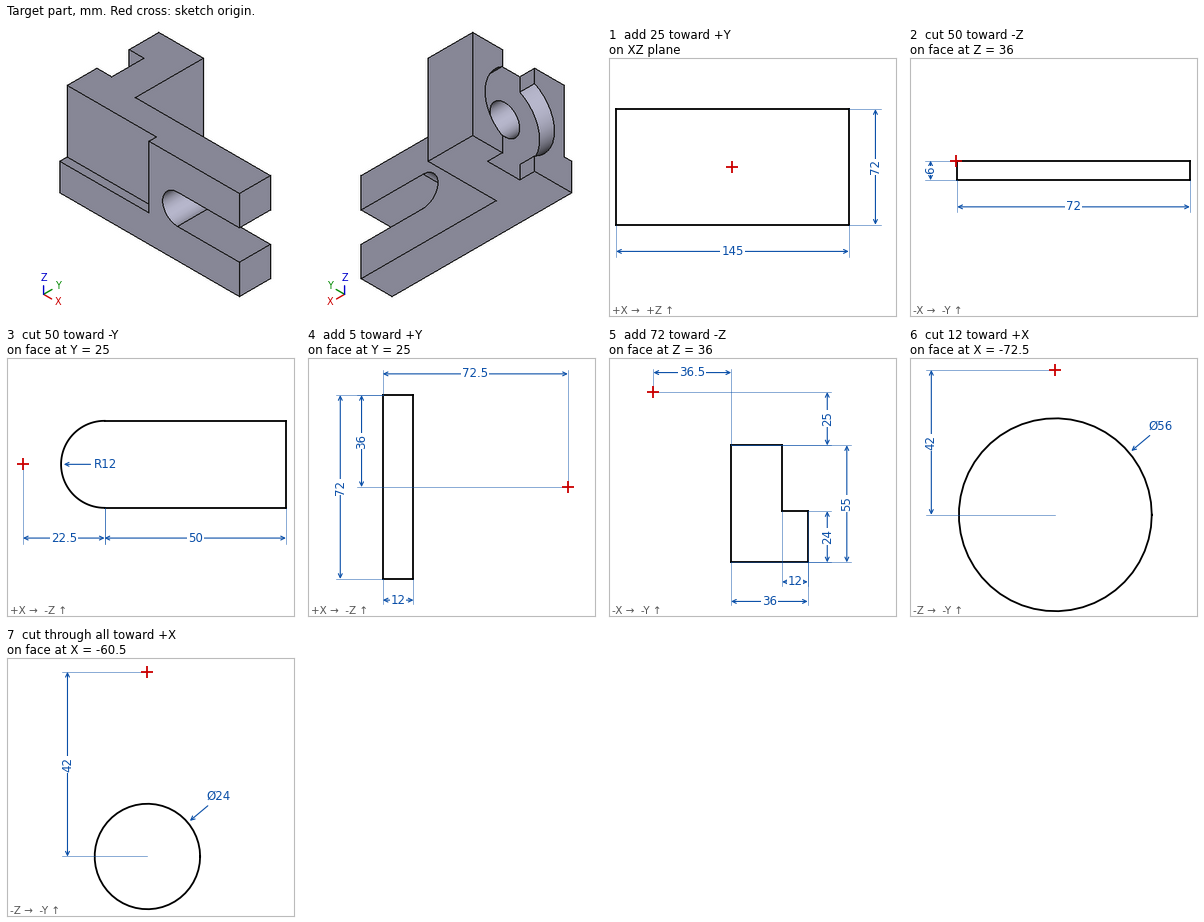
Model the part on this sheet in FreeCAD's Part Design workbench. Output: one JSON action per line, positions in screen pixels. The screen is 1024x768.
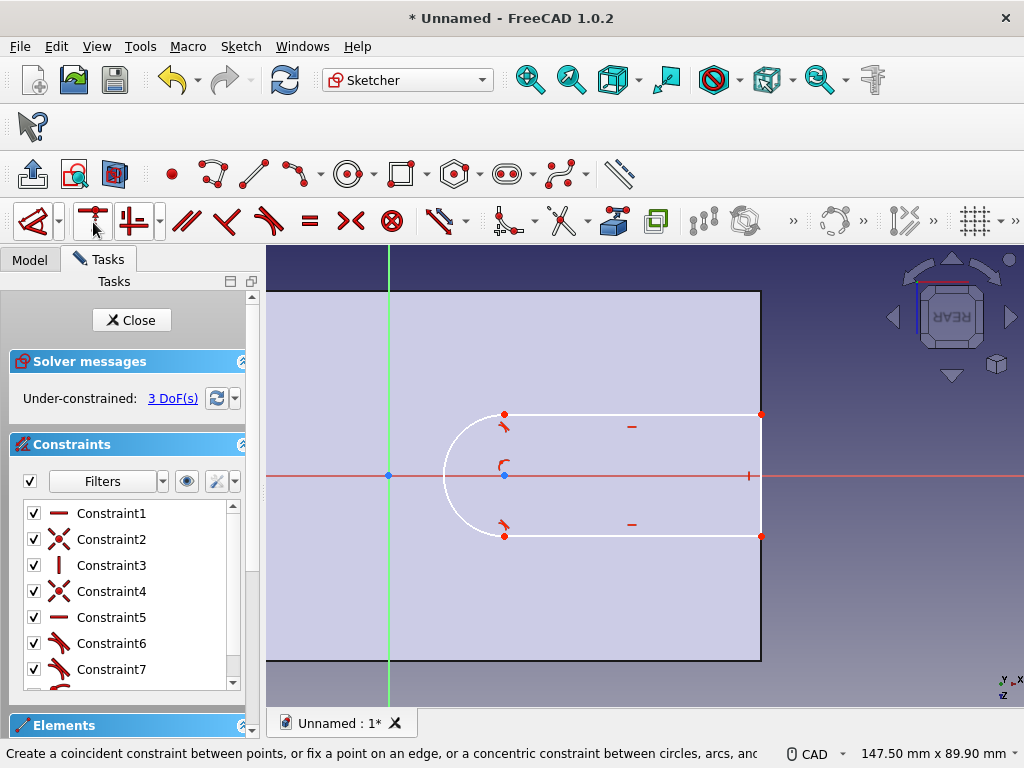
{"action": "left_click", "coordinate": [455, 440]}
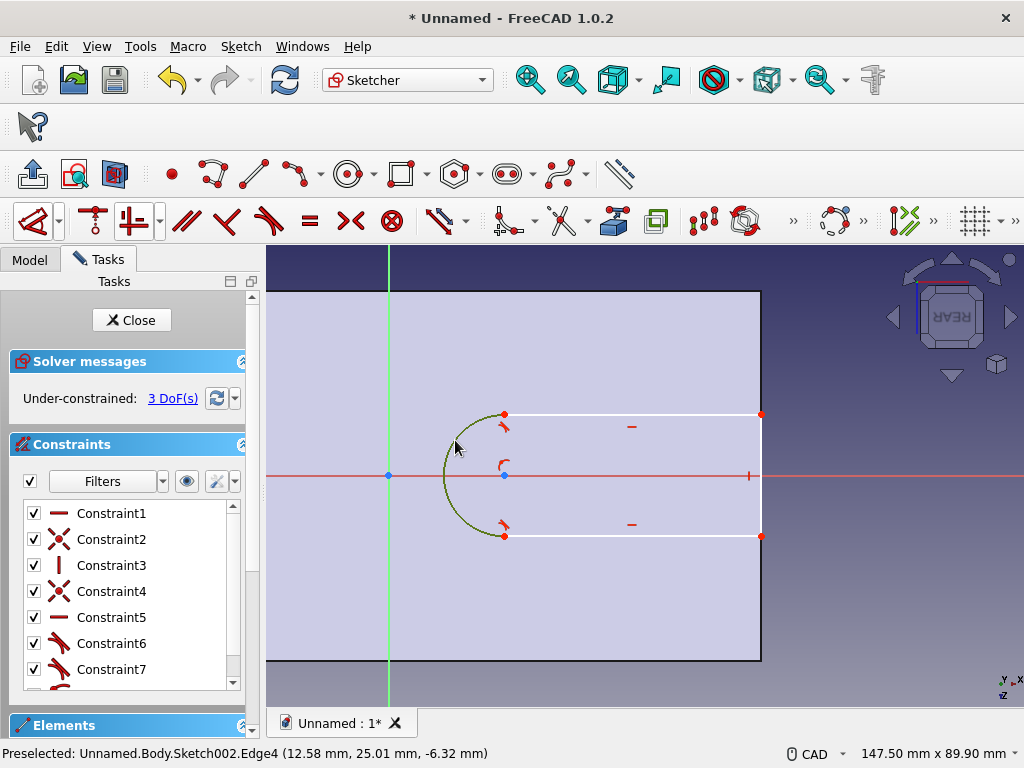
{"action": "left_click", "coordinate": [58, 222]}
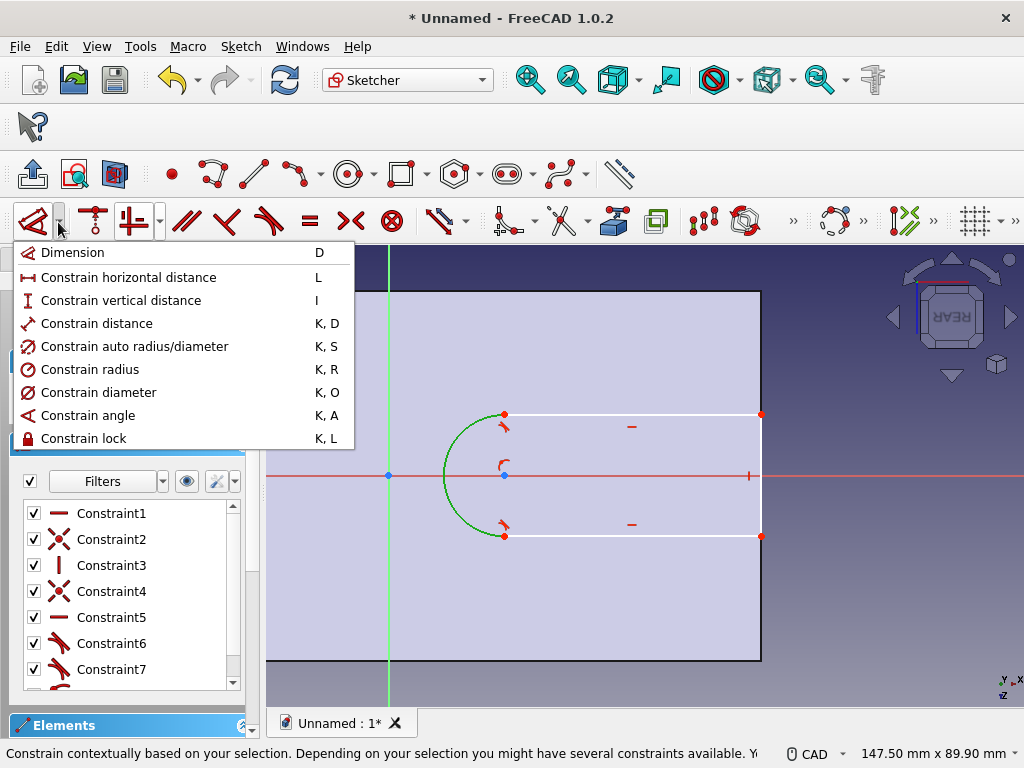
{"action": "left_click", "coordinate": [184, 370]}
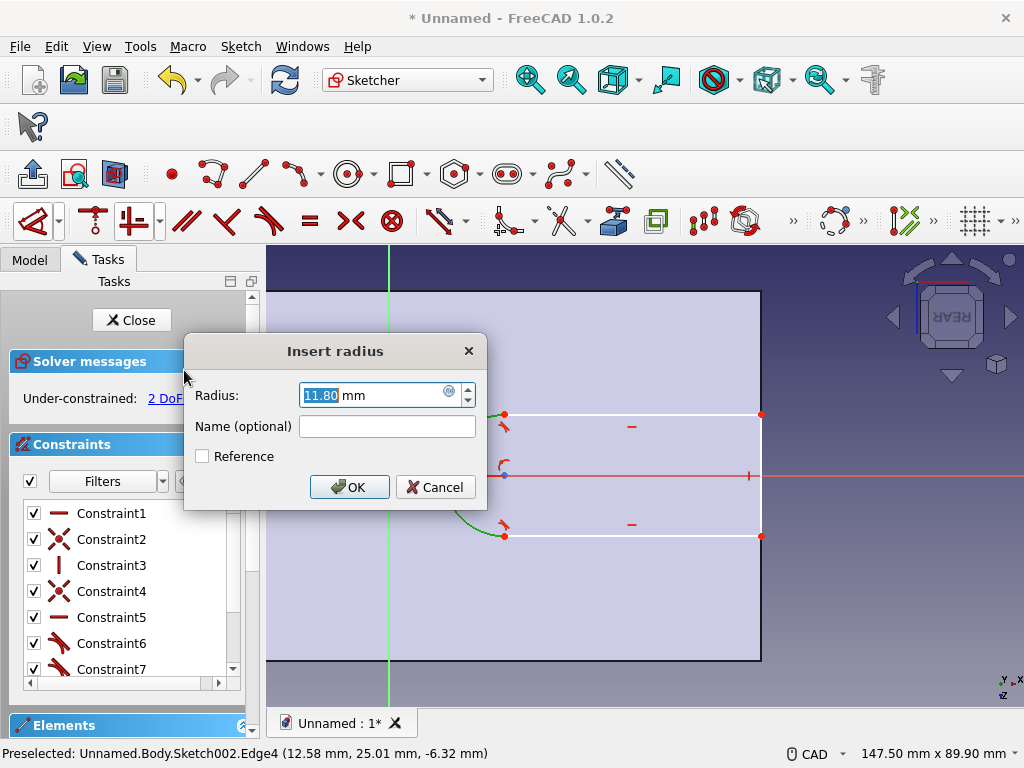
{"action": "type", "text": "12"}
{"action": "key", "text": "Return"}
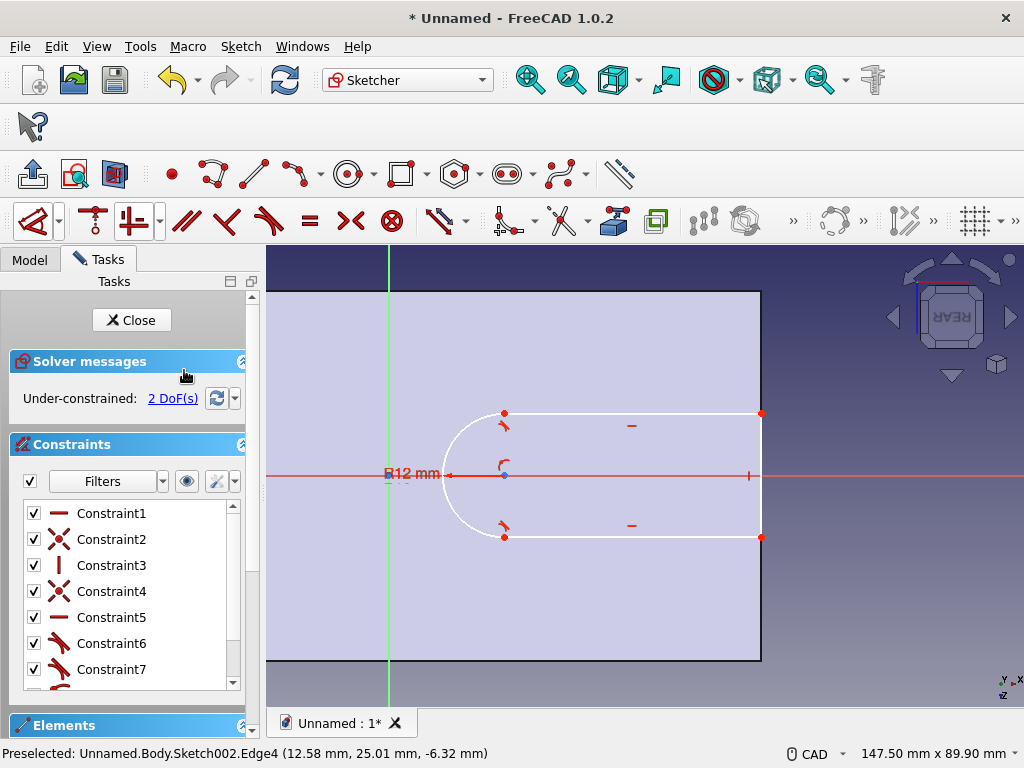
{"action": "left_click", "coordinate": [581, 537]}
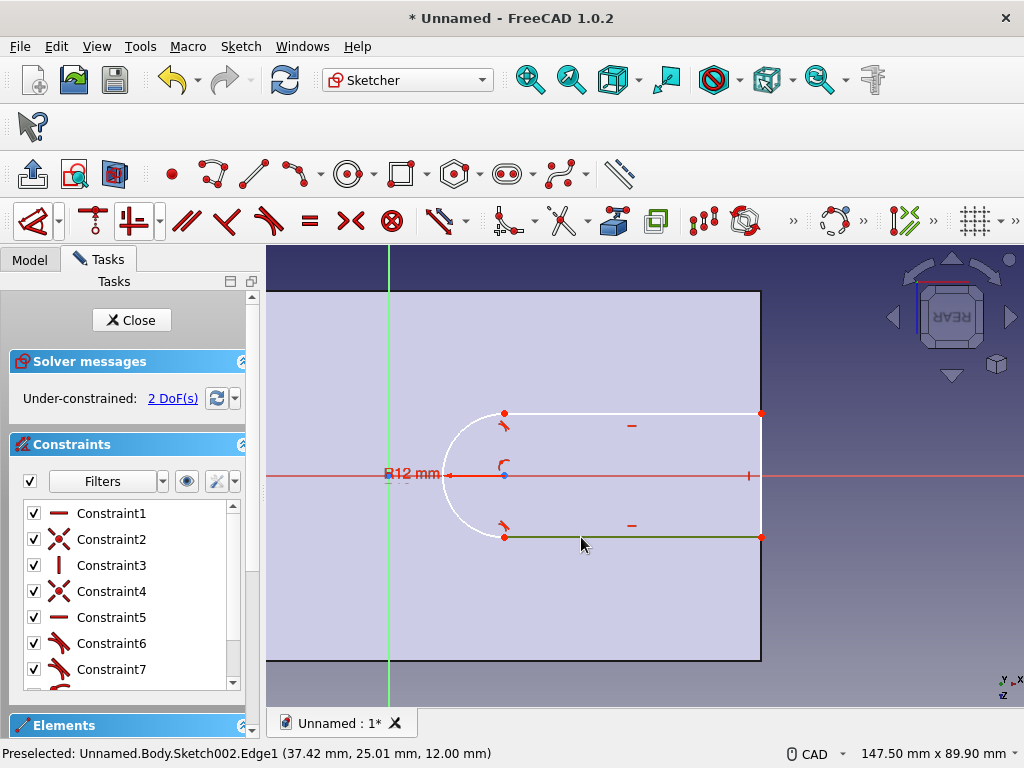
{"action": "left_click", "coordinate": [58, 222]}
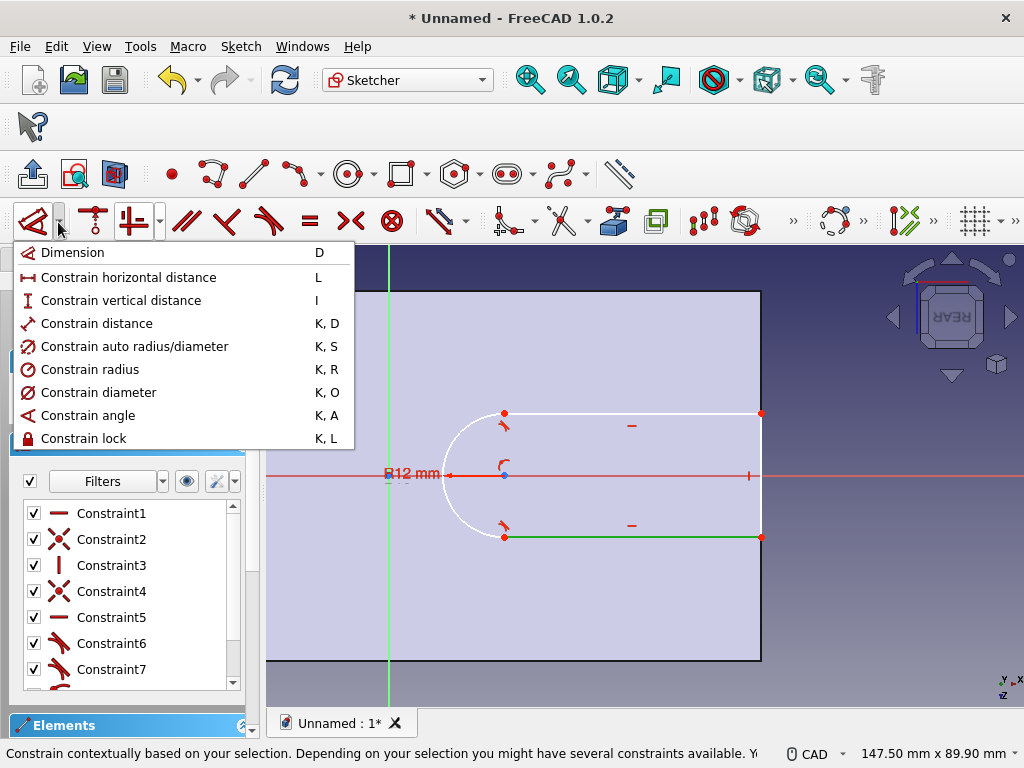
{"action": "left_click", "coordinate": [184, 278]}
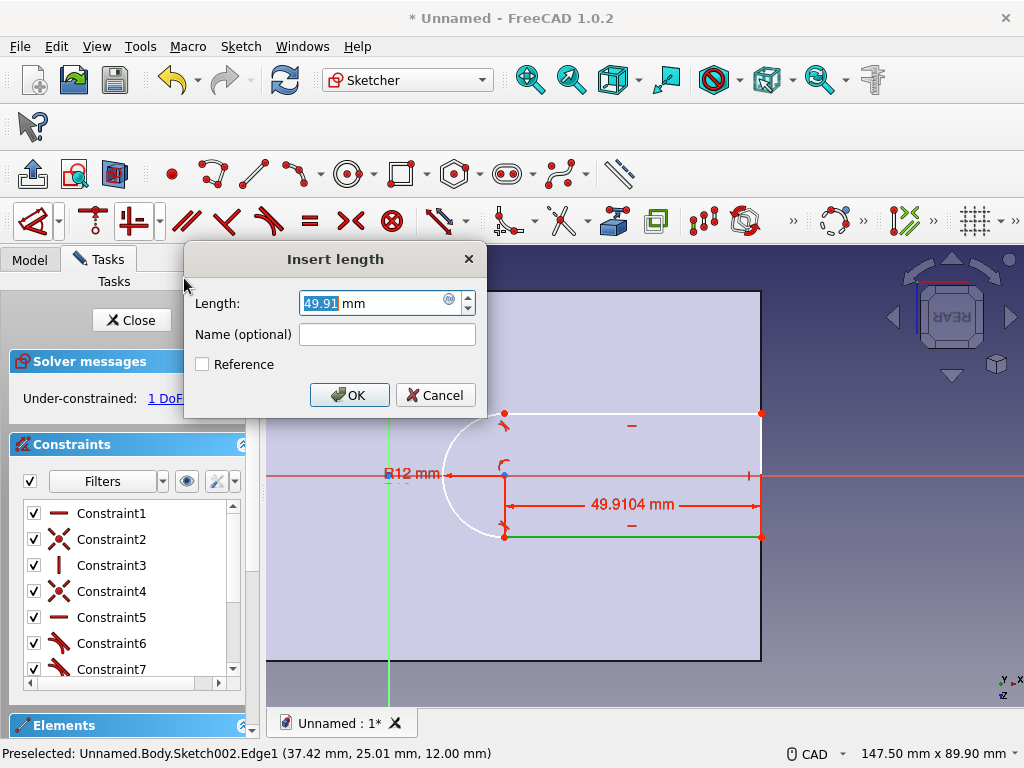
{"action": "type", "text": "50"}
{"action": "key", "text": "Return"}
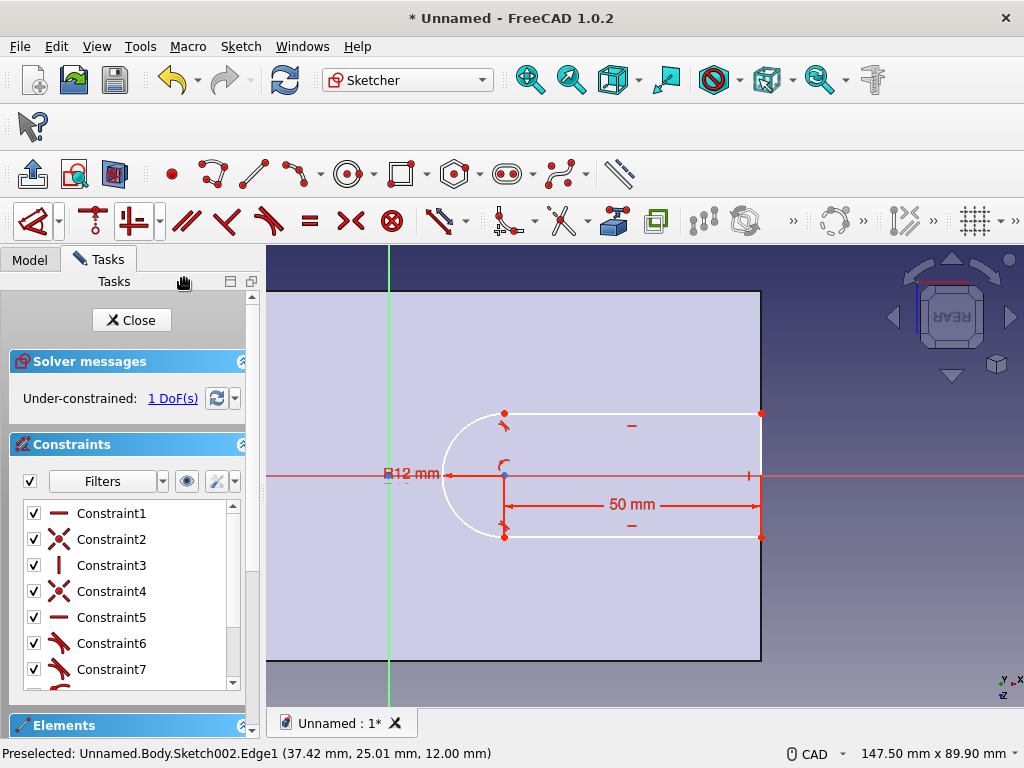
{"action": "left_click", "coordinate": [504, 537]}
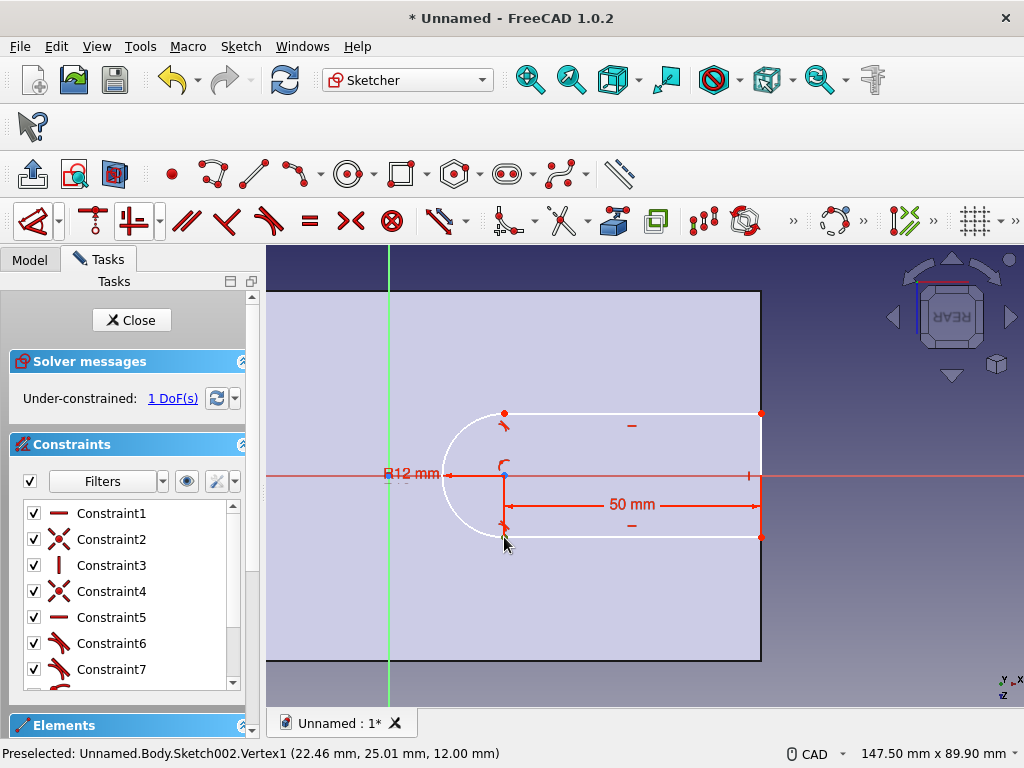
{"action": "left_click", "coordinate": [58, 222]}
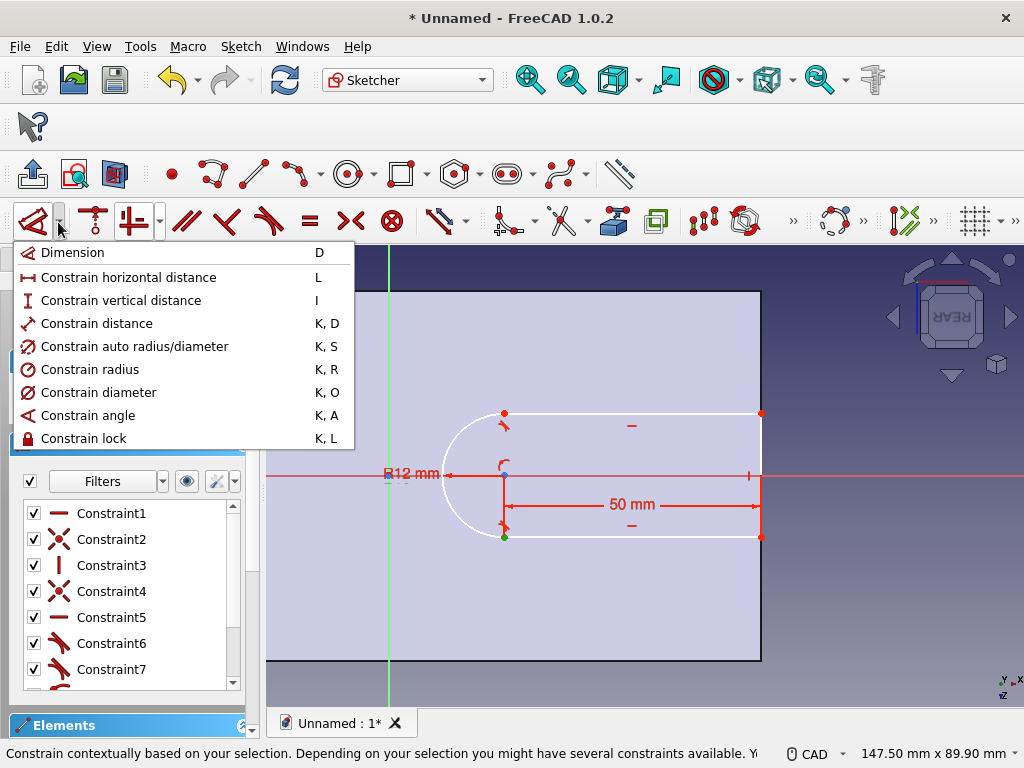
{"action": "left_click", "coordinate": [184, 278]}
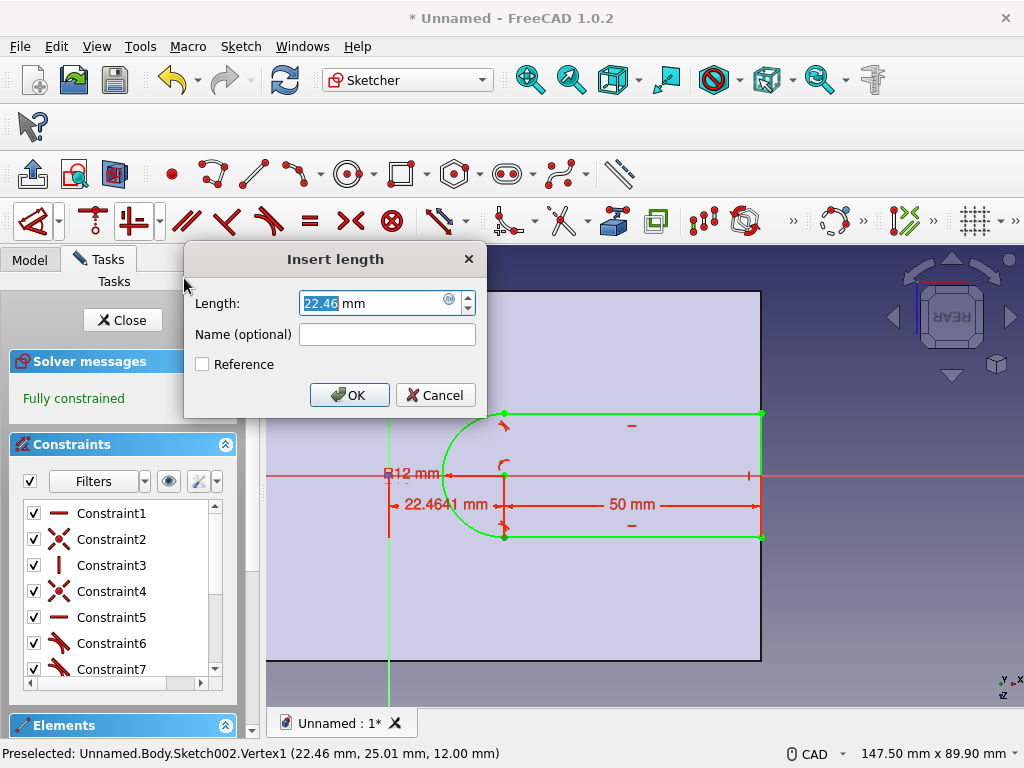
{"action": "type", "text": "22.5"}
{"action": "key", "text": "Return"}